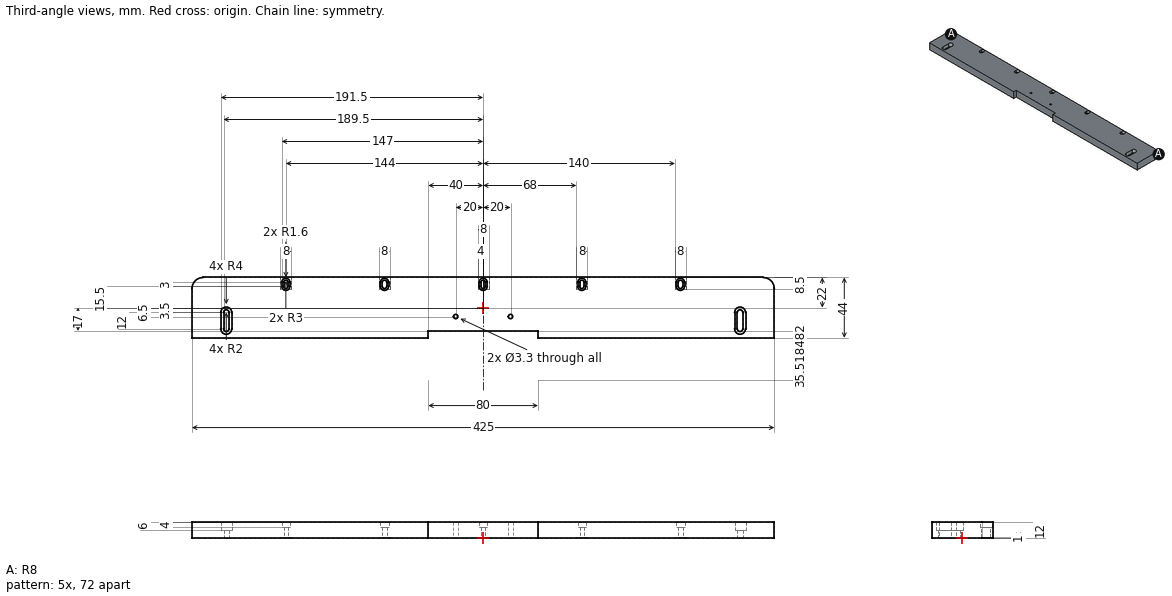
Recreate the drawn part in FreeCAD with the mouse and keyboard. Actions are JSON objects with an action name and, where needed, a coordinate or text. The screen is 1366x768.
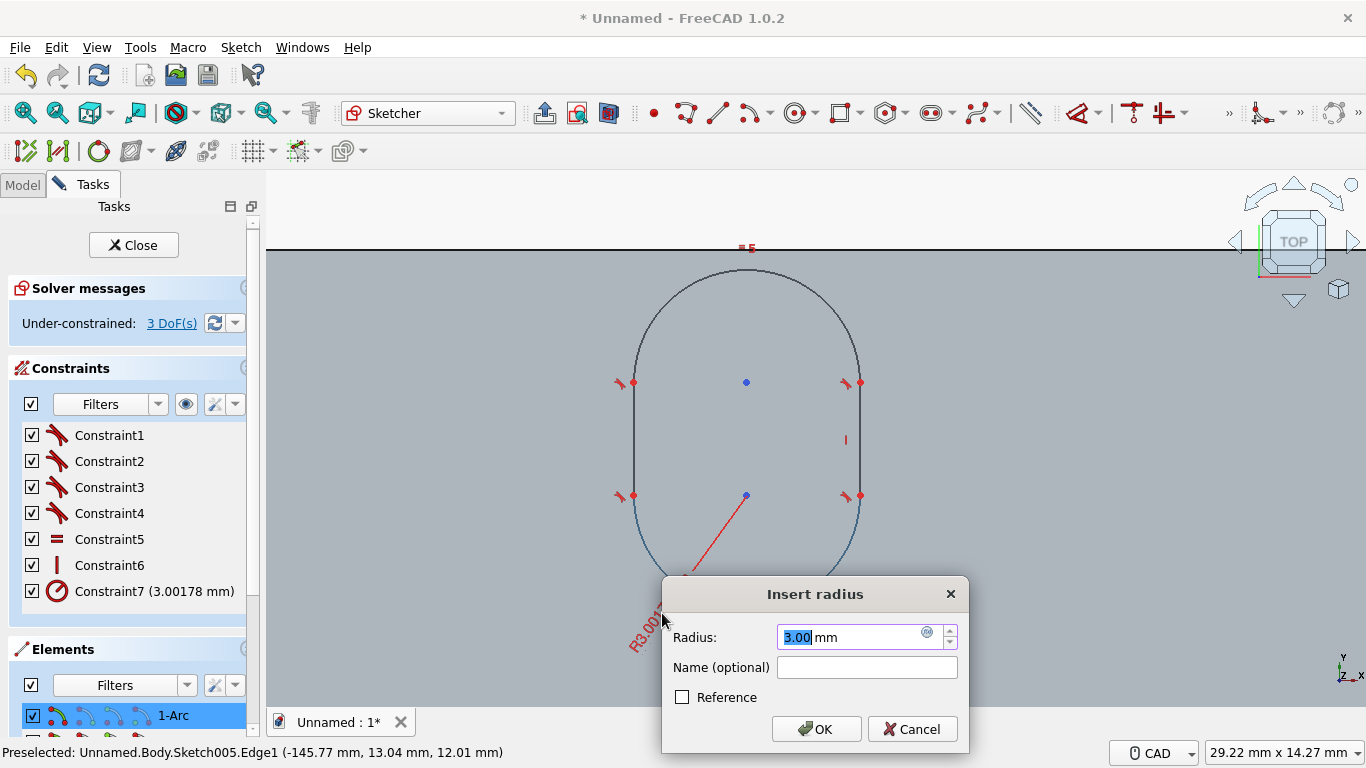
{"action": "type", "text": "3"}
{"action": "key", "text": "Return"}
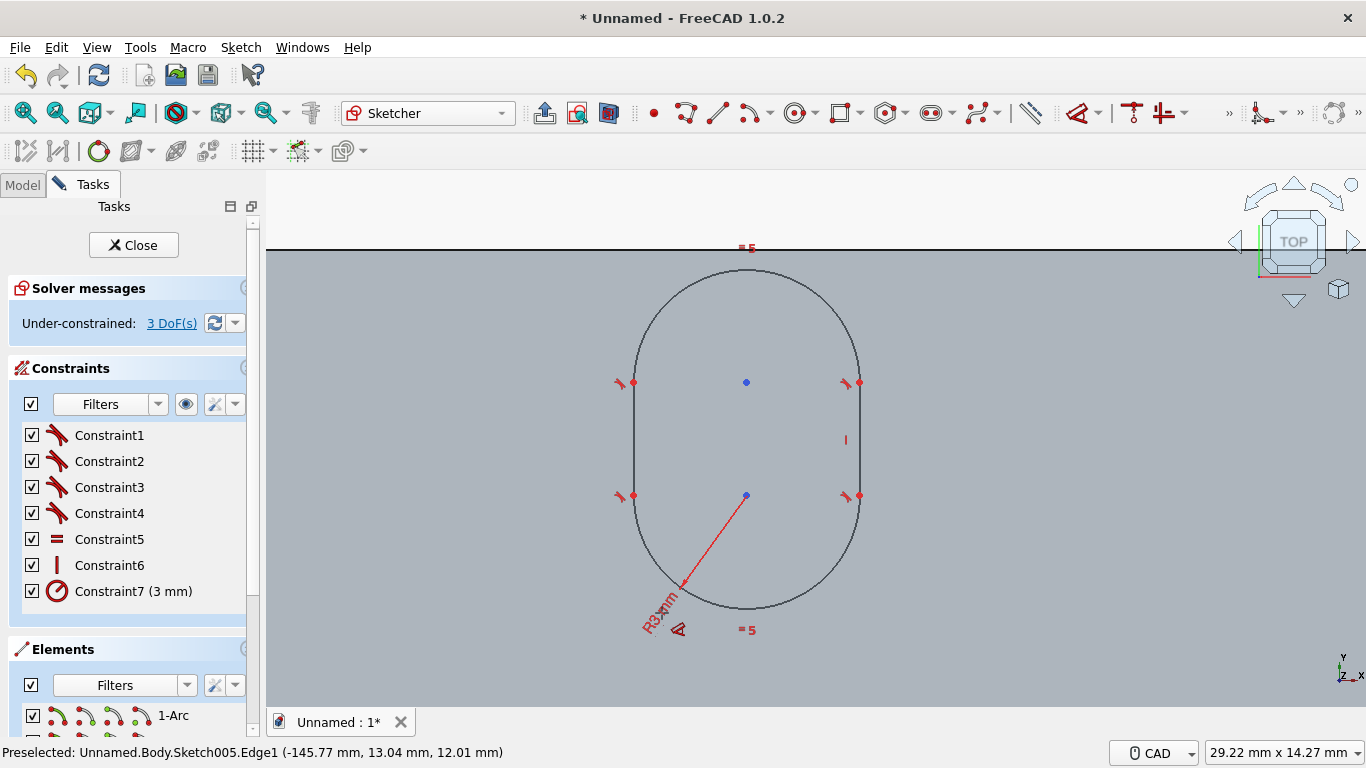
{"action": "left_click", "coordinate": [634, 462]}
{"action": "left_click", "coordinate": [600, 440]}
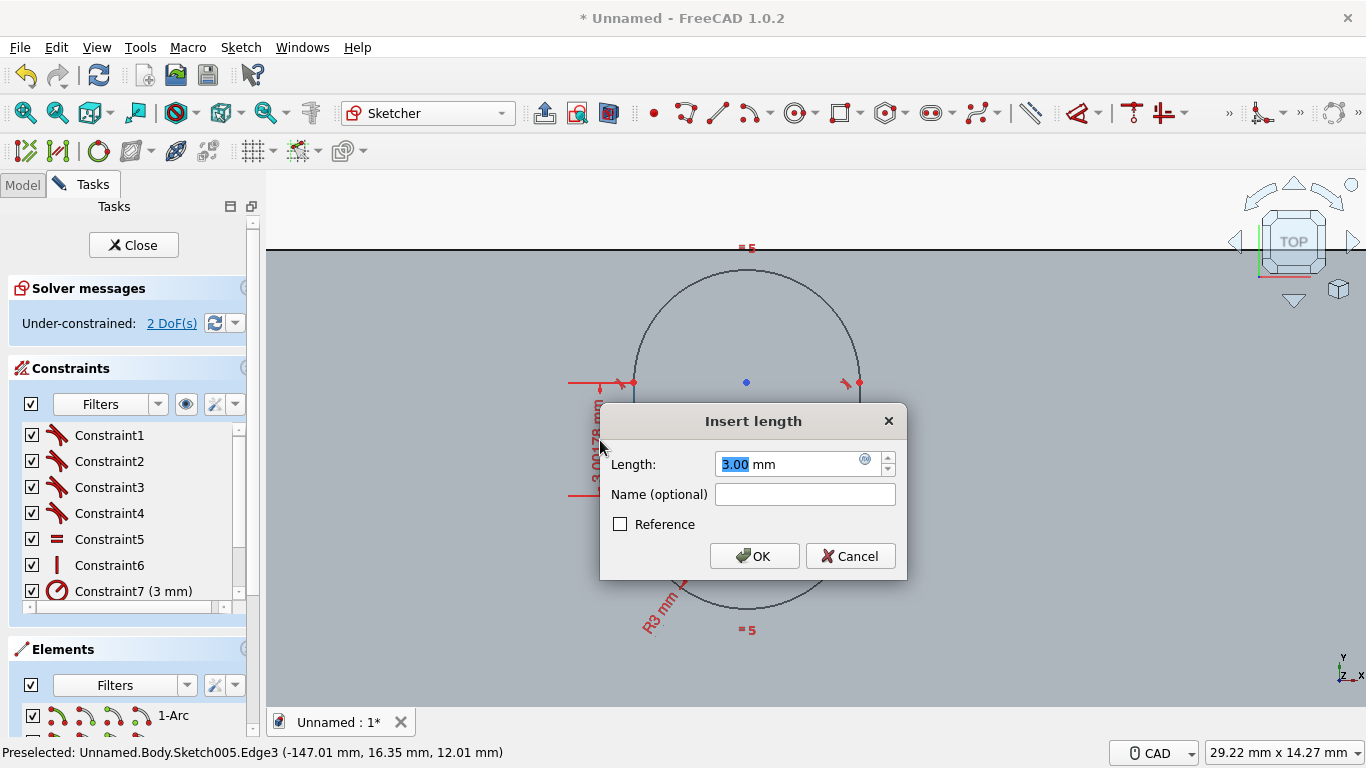
{"action": "type", "text": "3"}
{"action": "key", "text": "Return"}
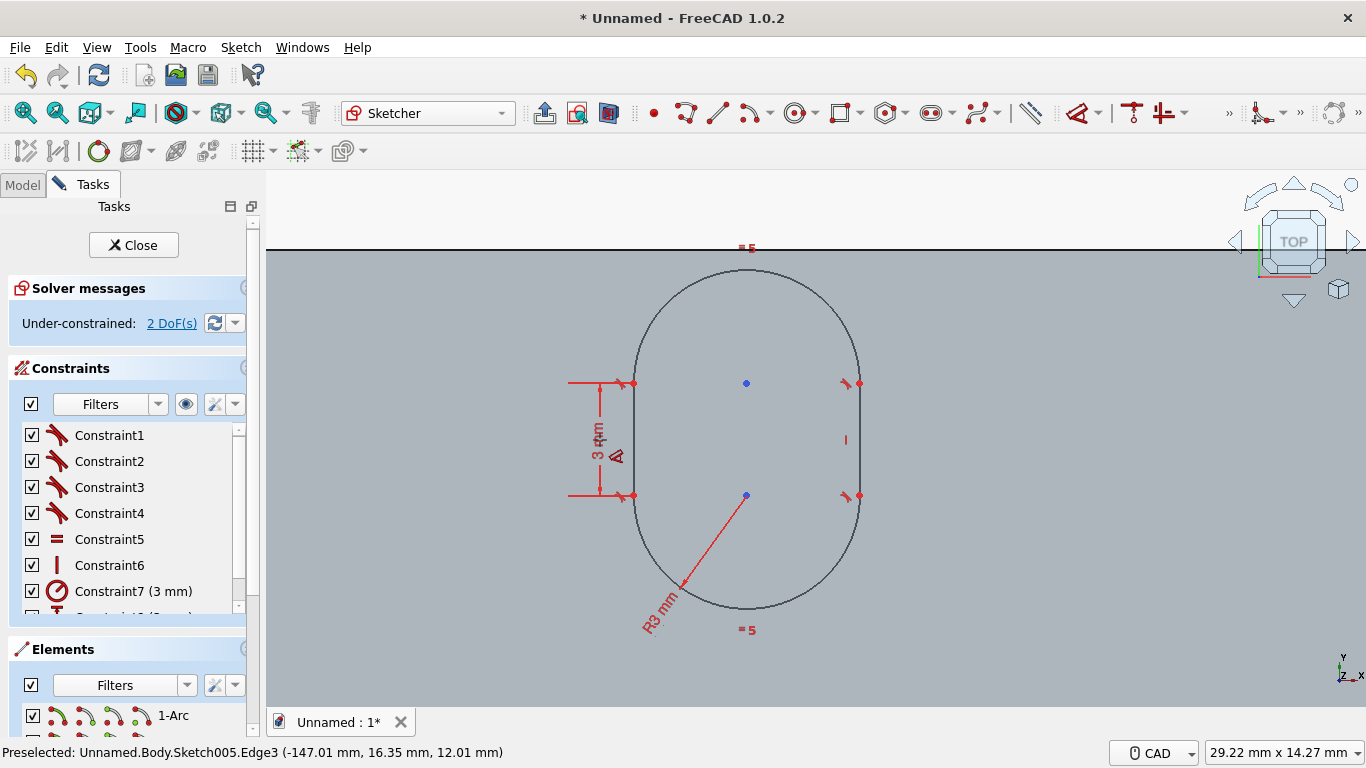
{"action": "left_click", "coordinate": [634, 496]}
{"action": "left_click", "coordinate": [917, 462]}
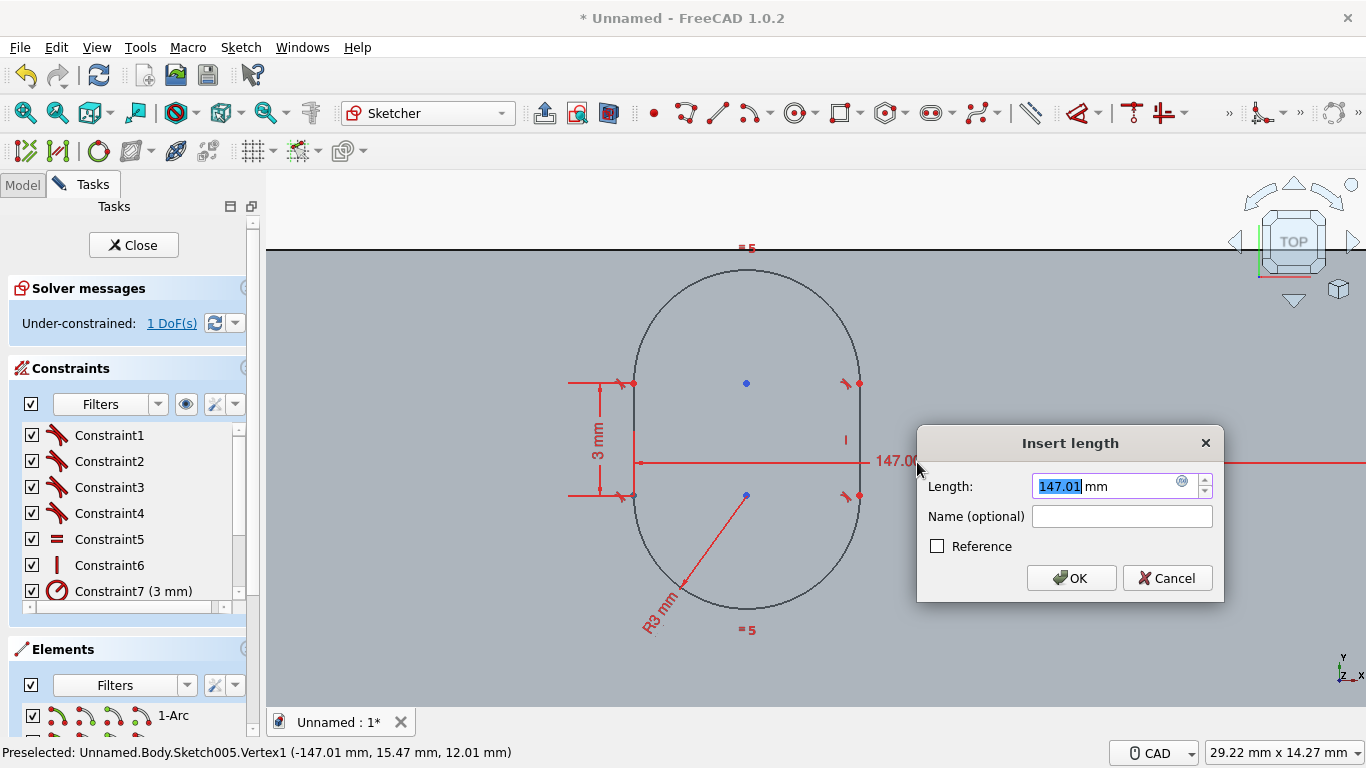
{"action": "type", "text": "147"}
{"action": "key", "text": "Return"}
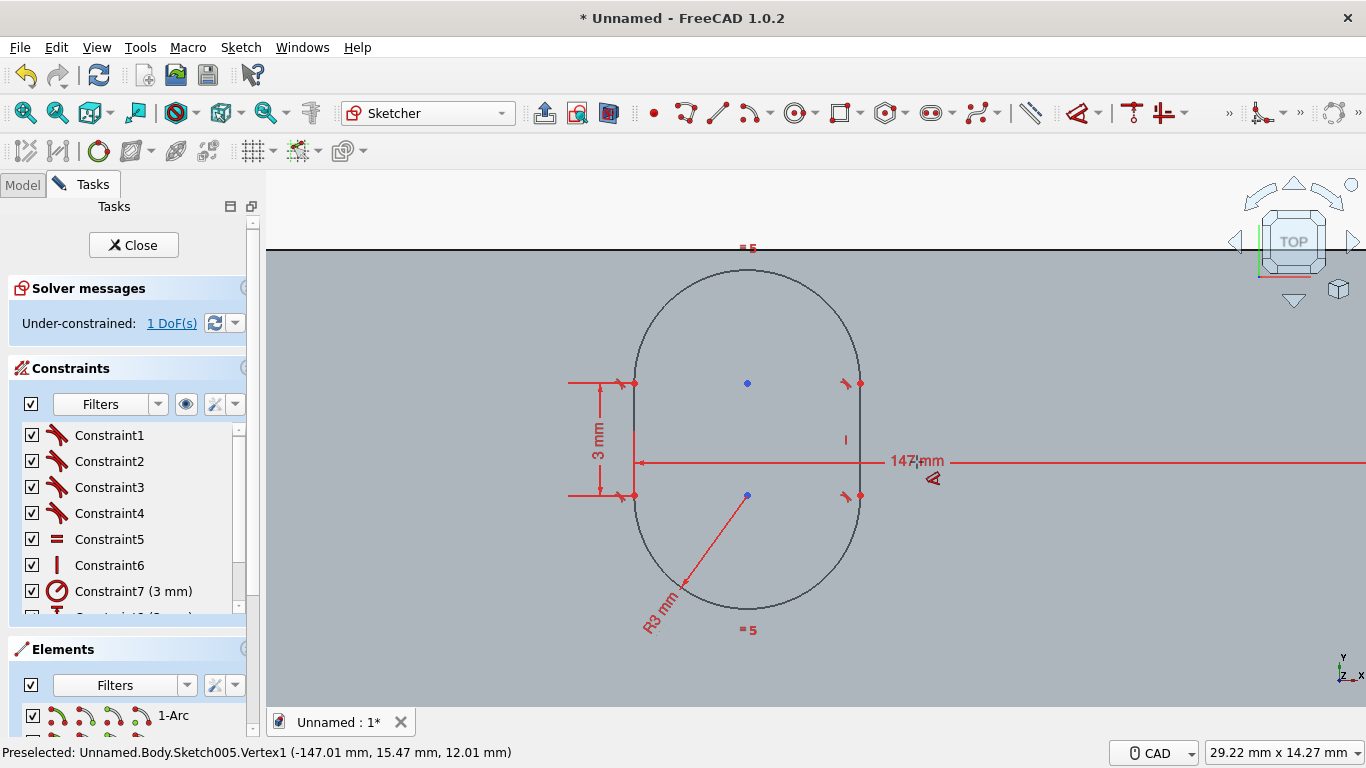
{"action": "left_click", "coordinate": [634, 496]}
{"action": "left_click", "coordinate": [600, 588]}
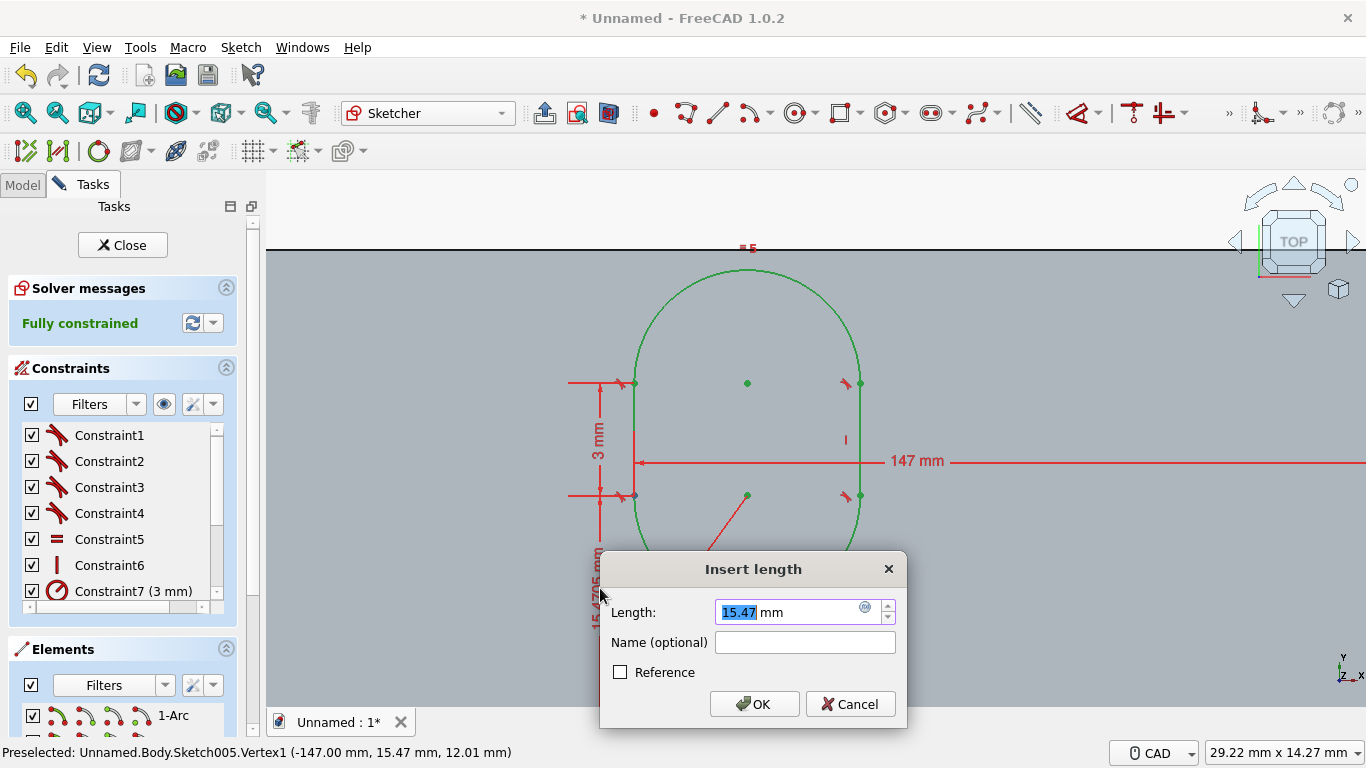
{"action": "type", "text": "15.5"}
{"action": "key", "text": "Return"}
{"action": "key", "text": "Escape"}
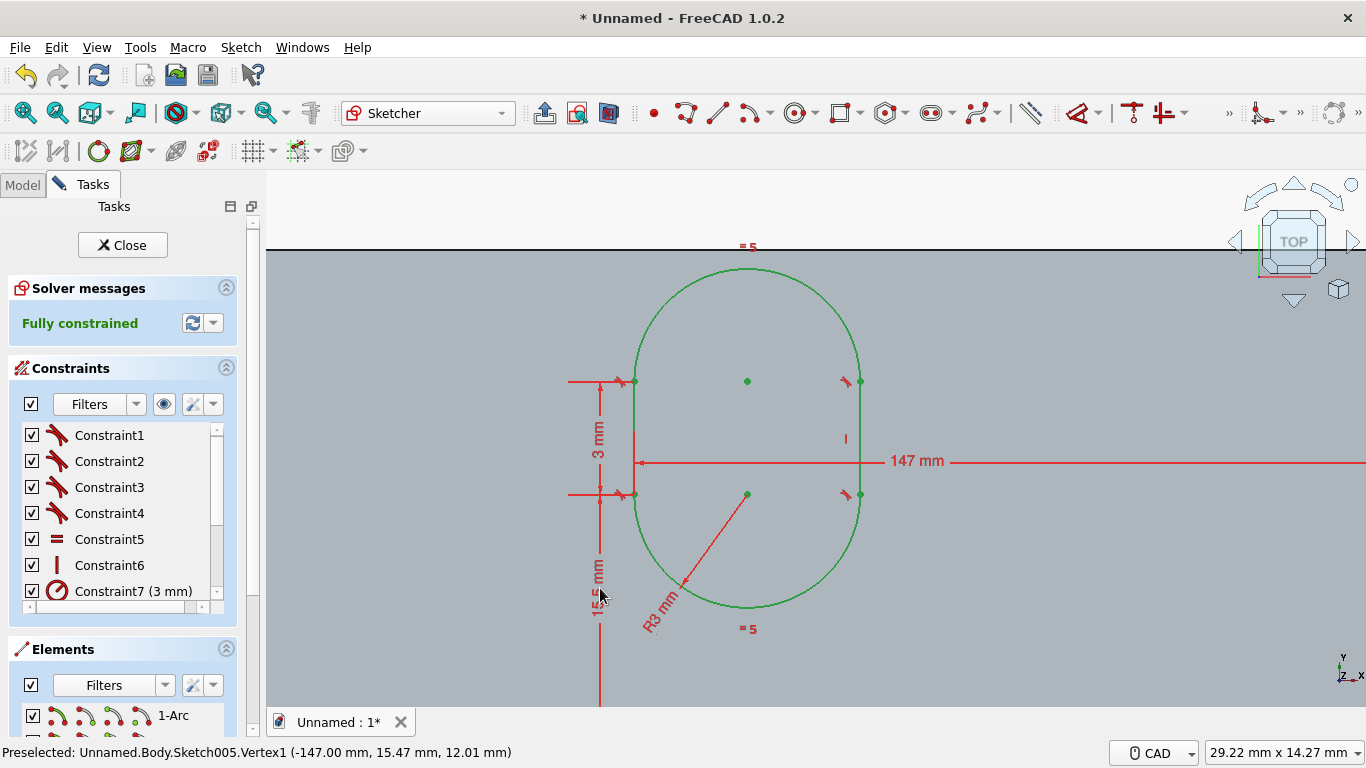
{"action": "left_click", "coordinate": [123, 245]}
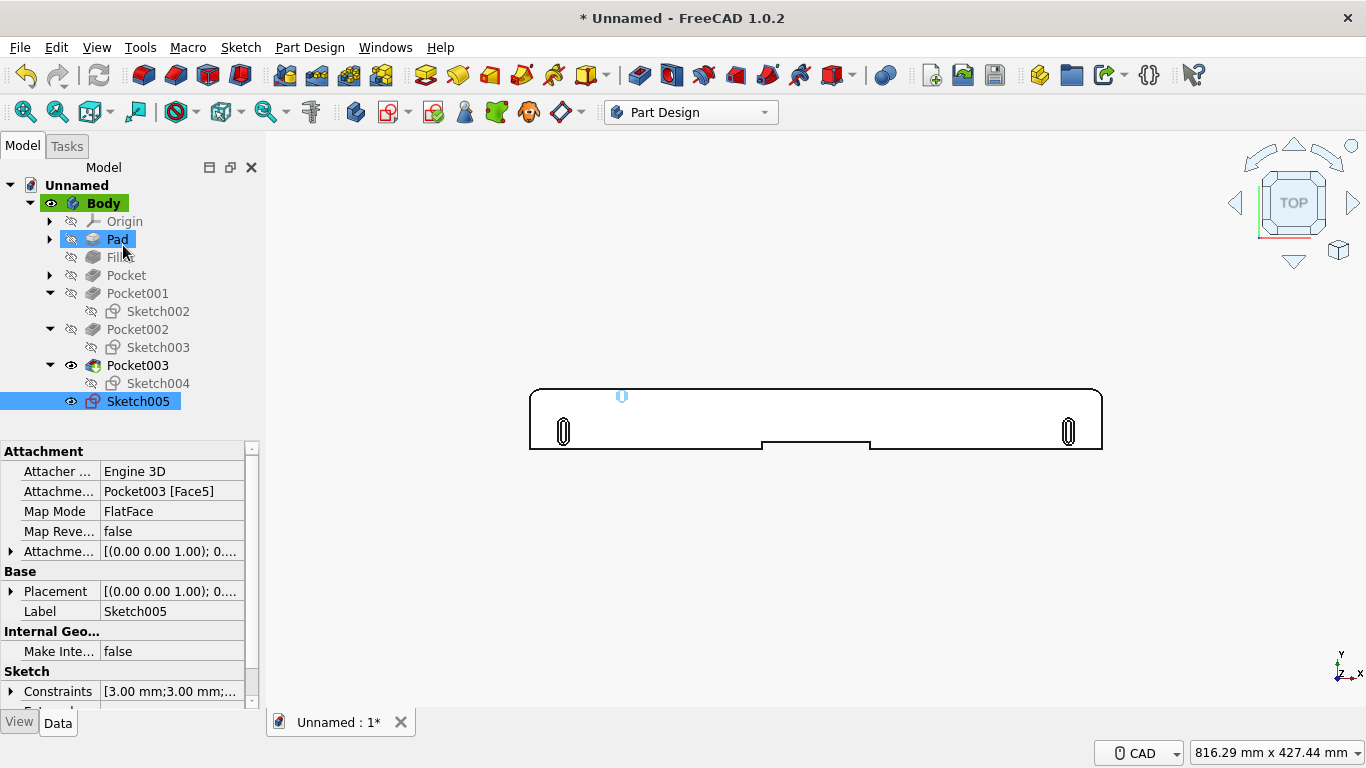
{"action": "left_click", "coordinate": [640, 76]}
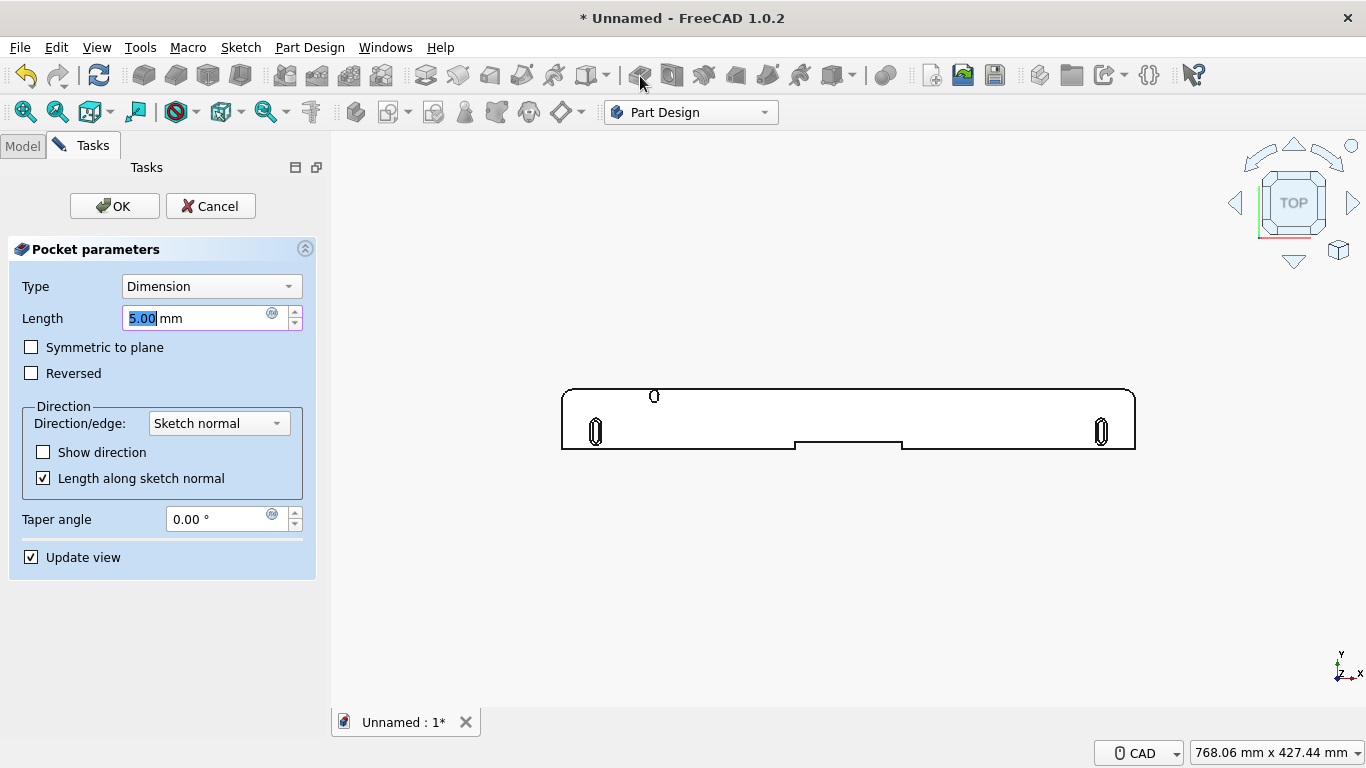
{"action": "type", "text": "4"}
{"action": "key", "text": "Tab"}